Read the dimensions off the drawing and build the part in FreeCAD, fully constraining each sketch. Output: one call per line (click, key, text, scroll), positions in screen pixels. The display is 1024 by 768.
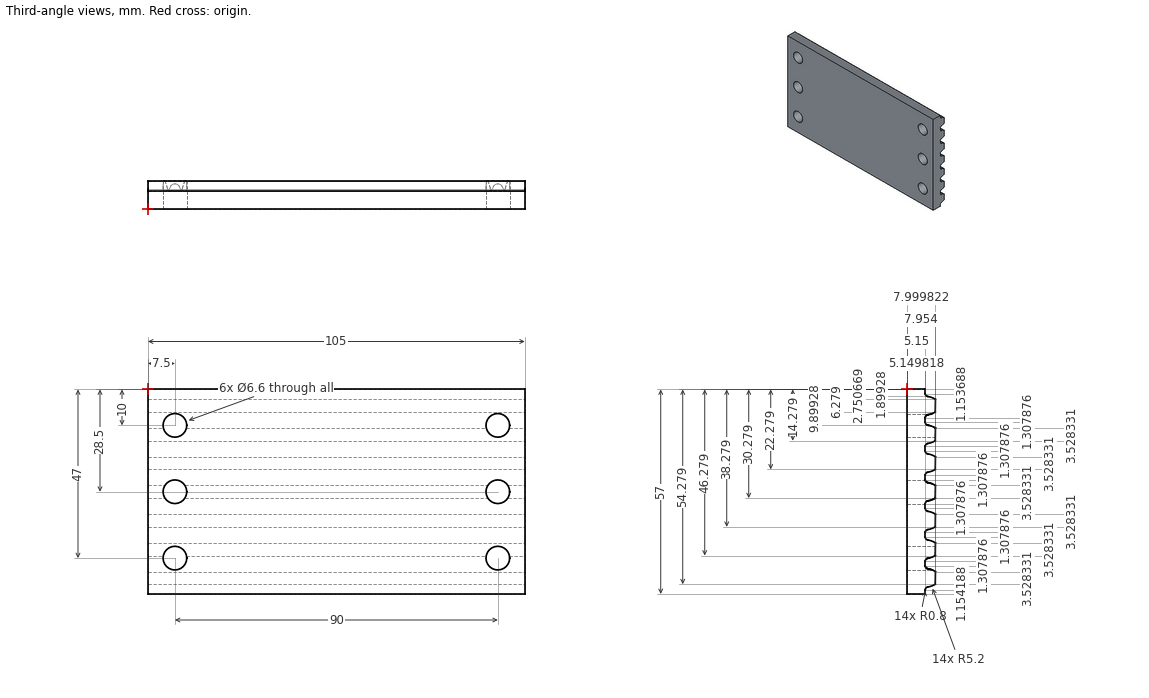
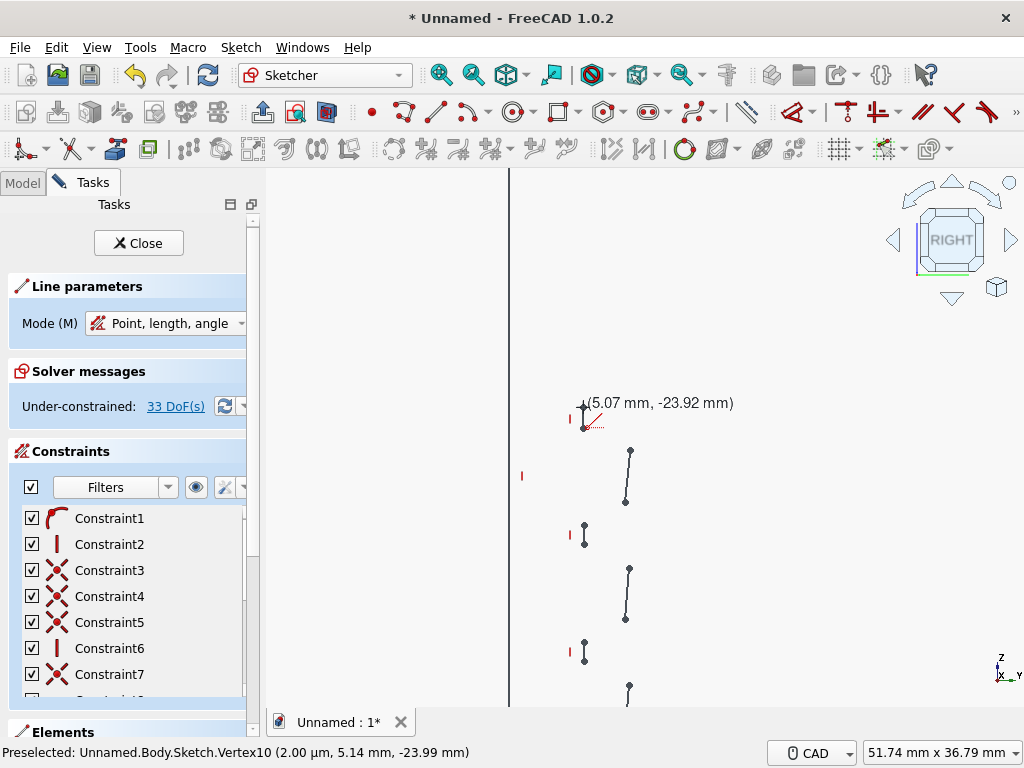
click(625, 384)
click(629, 332)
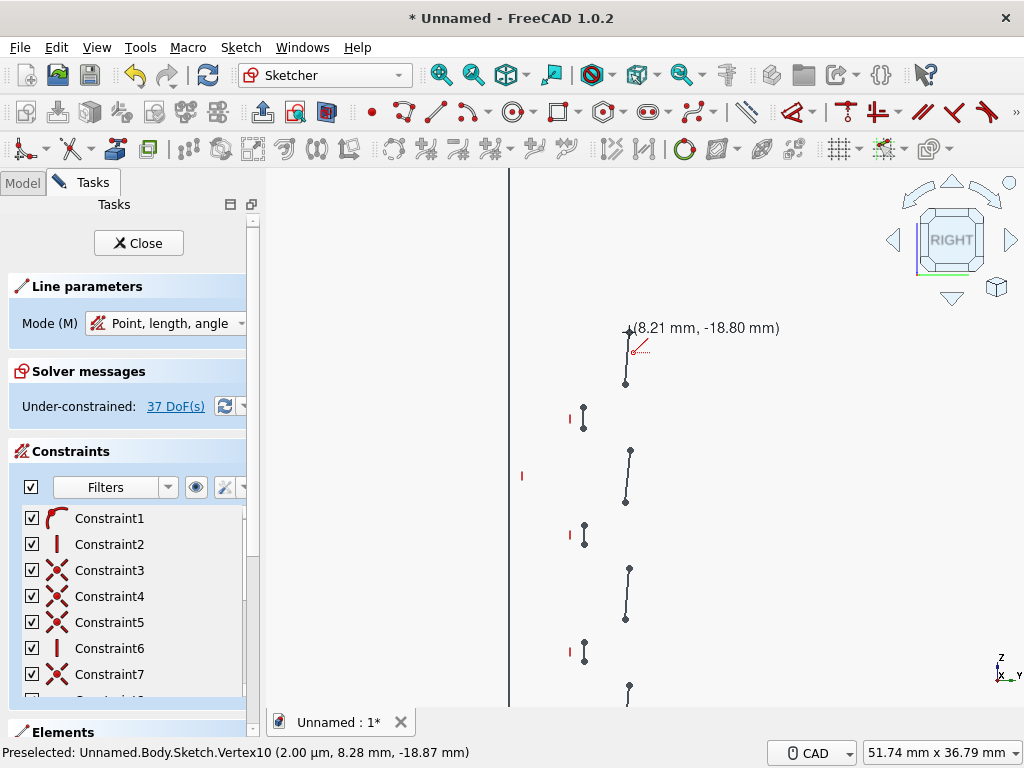
click(584, 309)
click(584, 290)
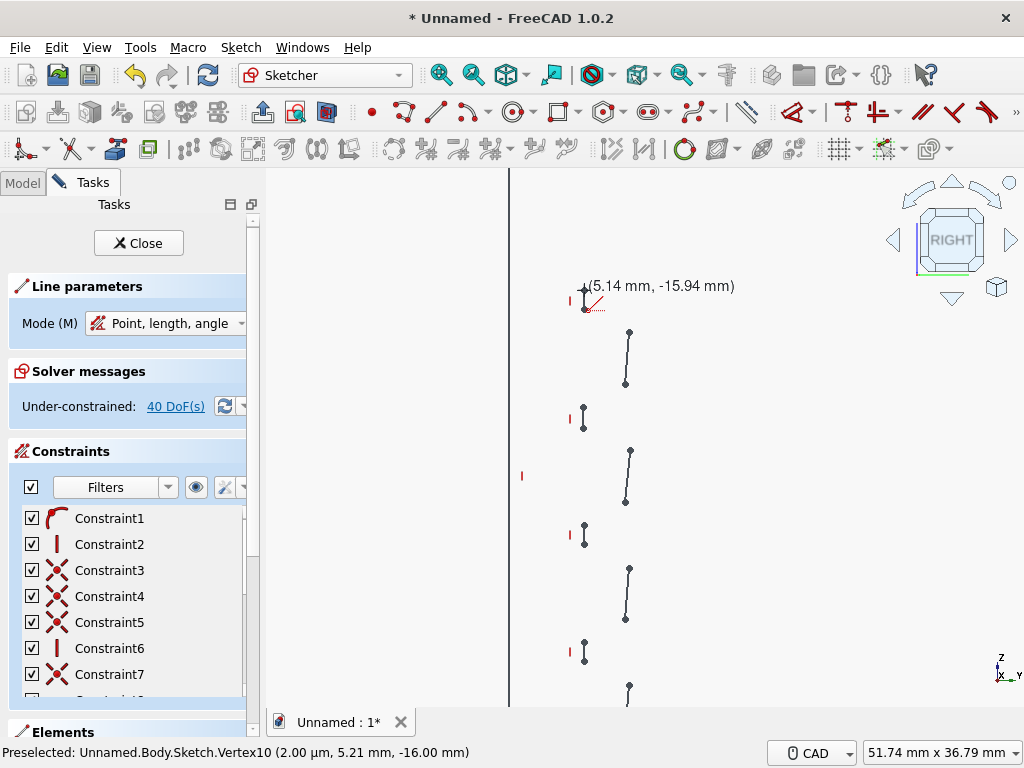
click(625, 267)
click(629, 215)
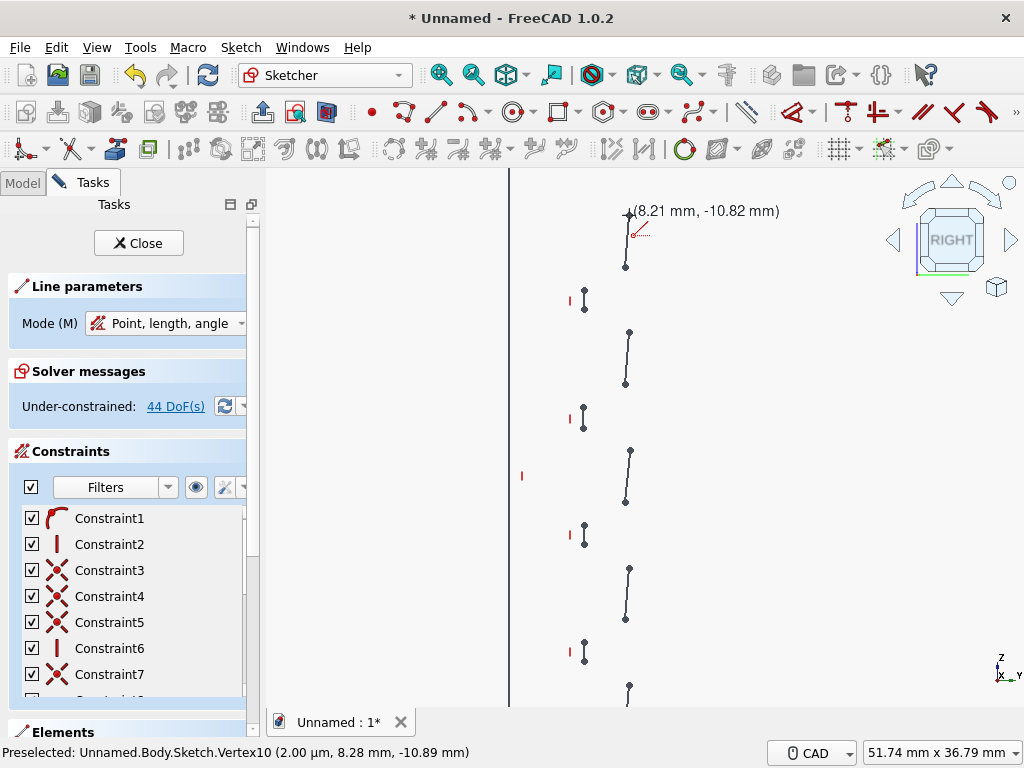
scroll(584, 407, down, 4)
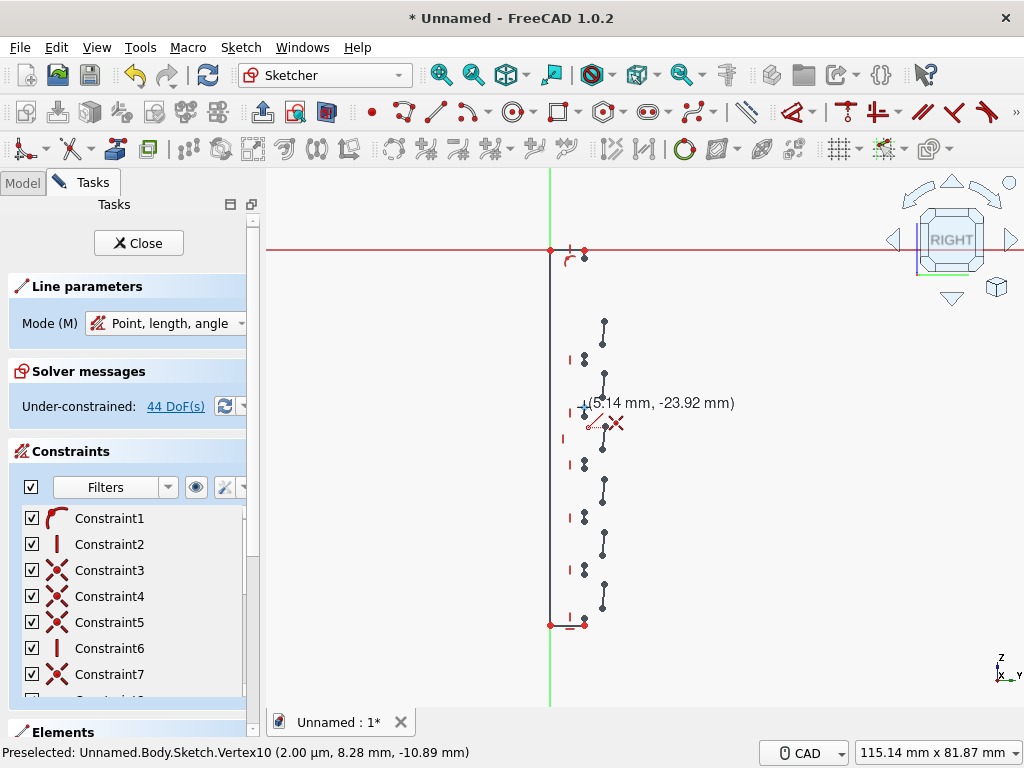
click(584, 310)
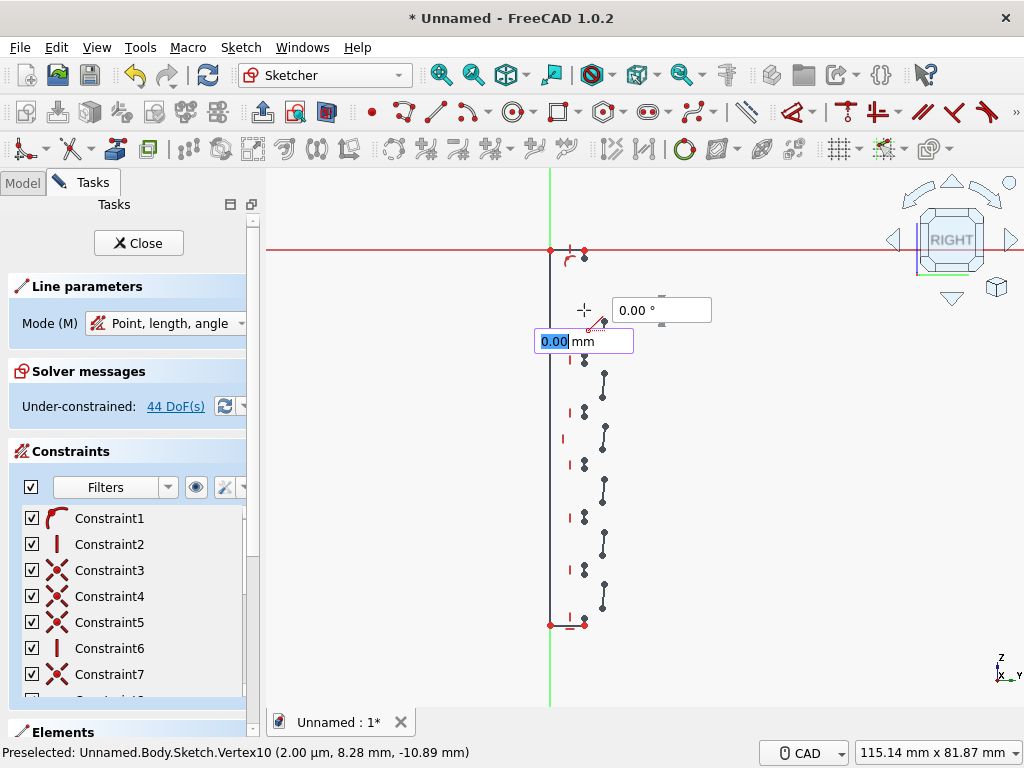
scroll(584, 302, up, 4)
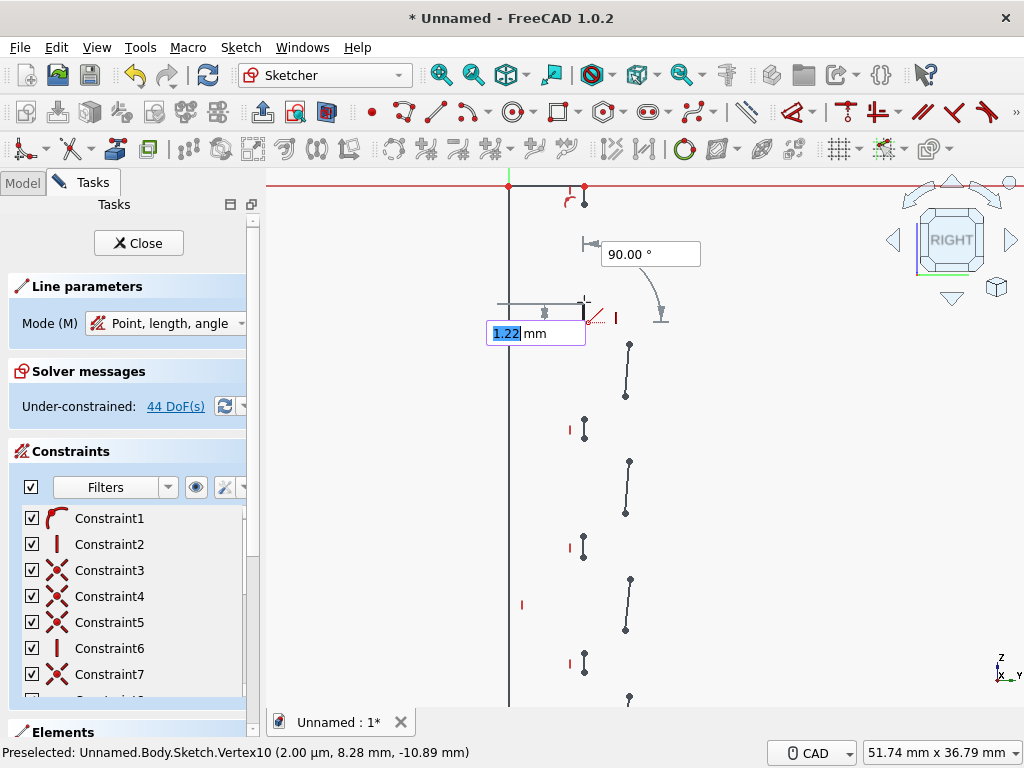
click(583, 301)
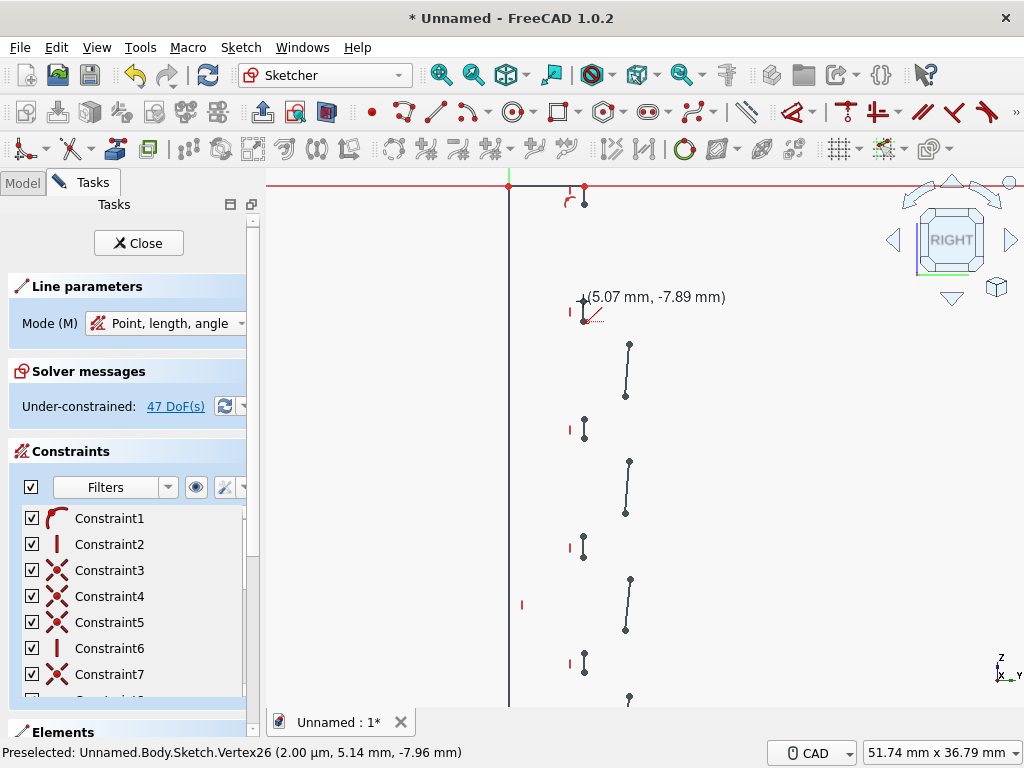
click(625, 278)
click(629, 227)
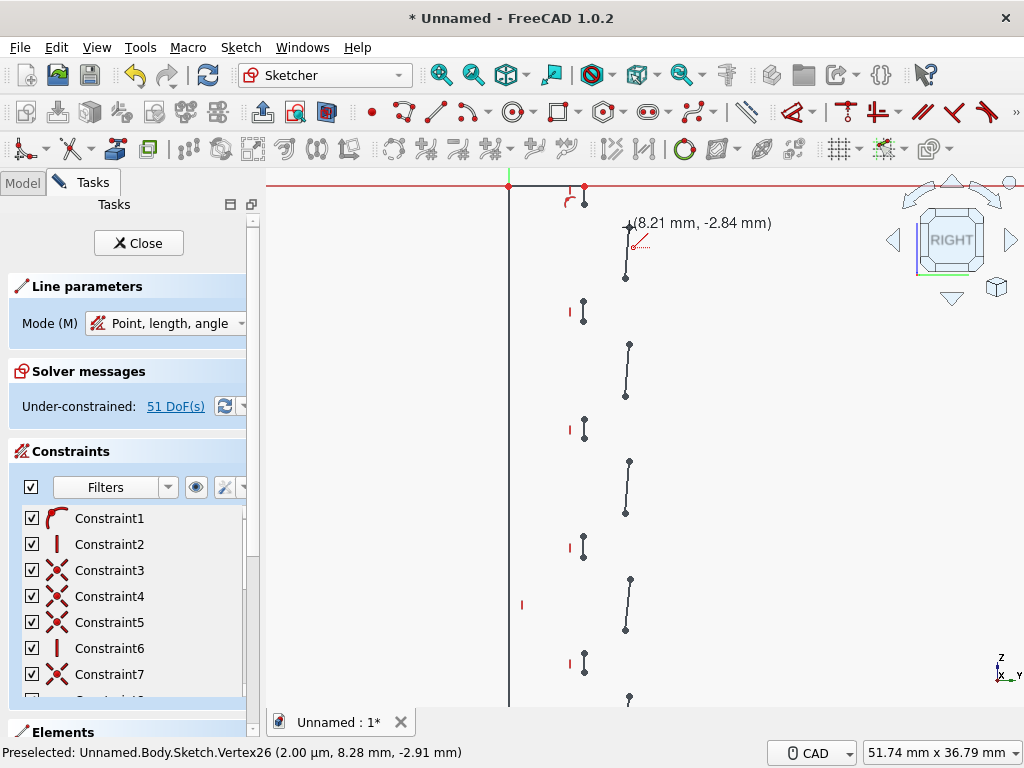
key(g)
key(3)
key(a)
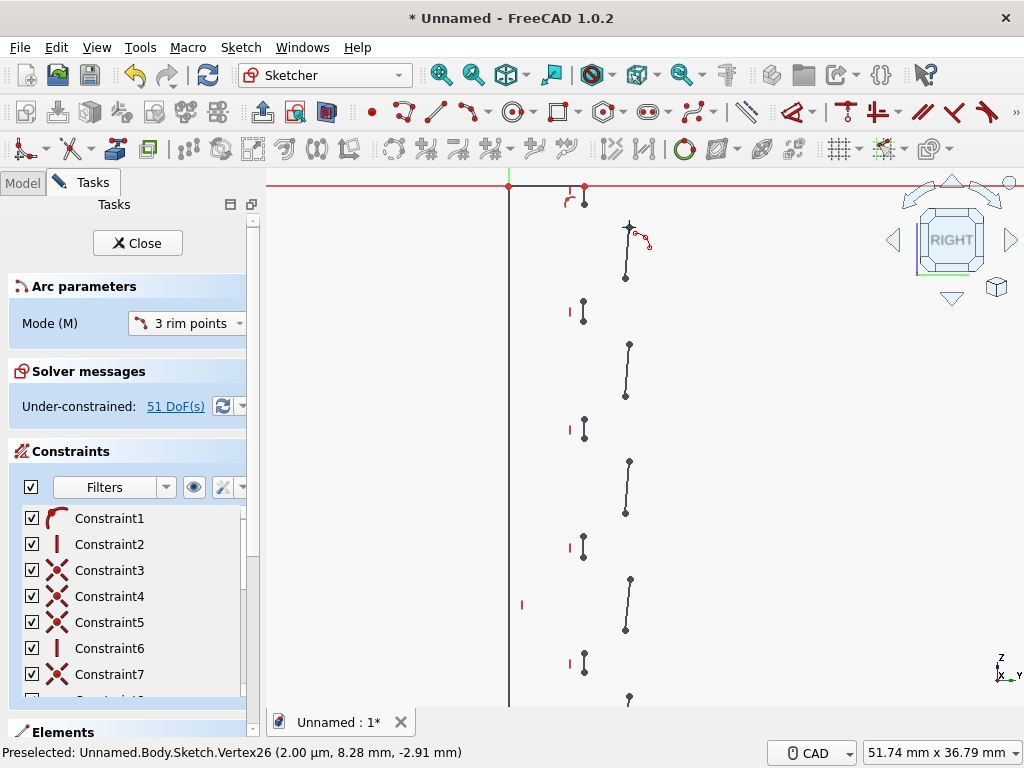
scroll(584, 302, down, 4)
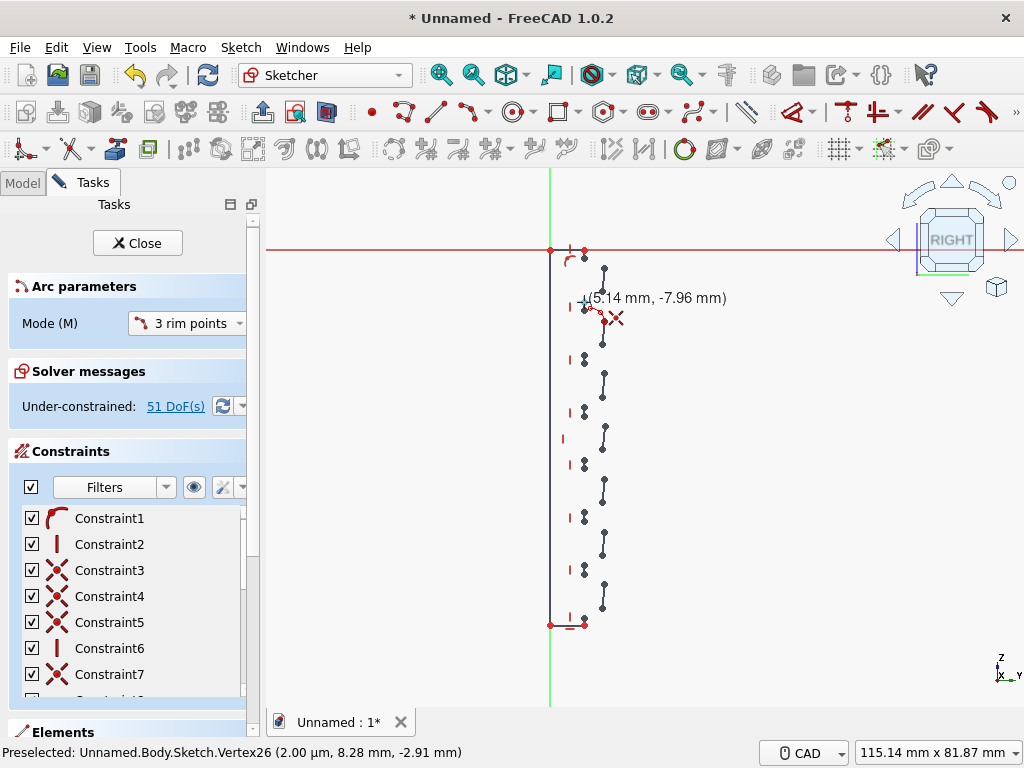
scroll(584, 618, up, 8)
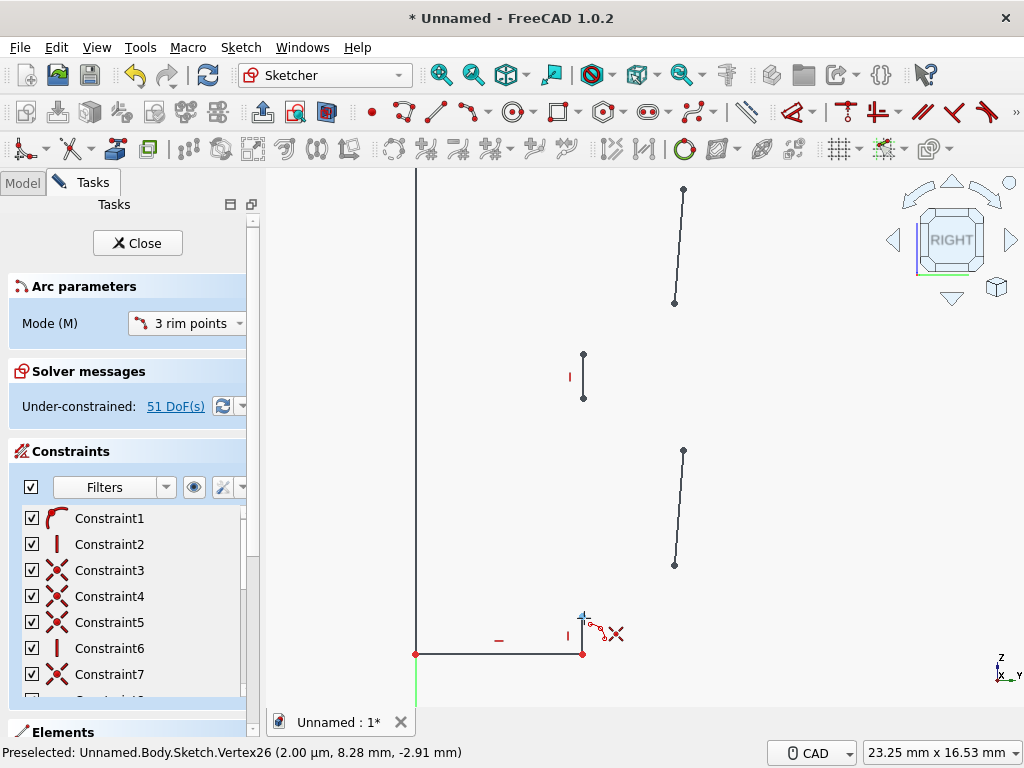
click(582, 617)
click(606, 588)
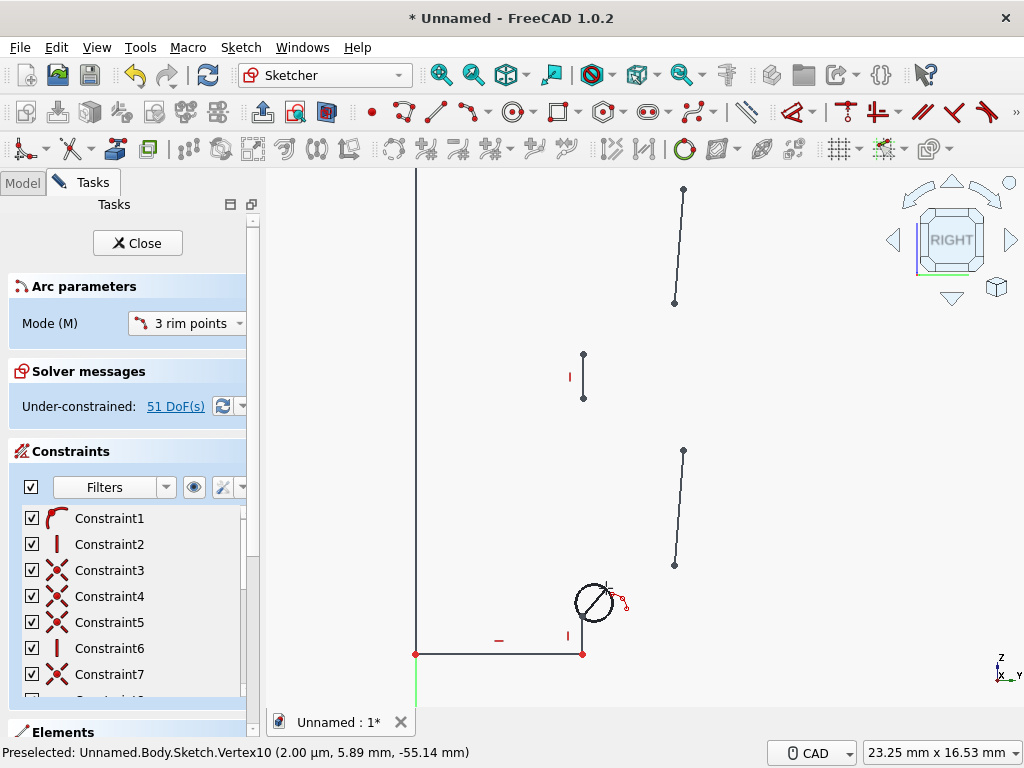
scroll(590, 597, up, 5)